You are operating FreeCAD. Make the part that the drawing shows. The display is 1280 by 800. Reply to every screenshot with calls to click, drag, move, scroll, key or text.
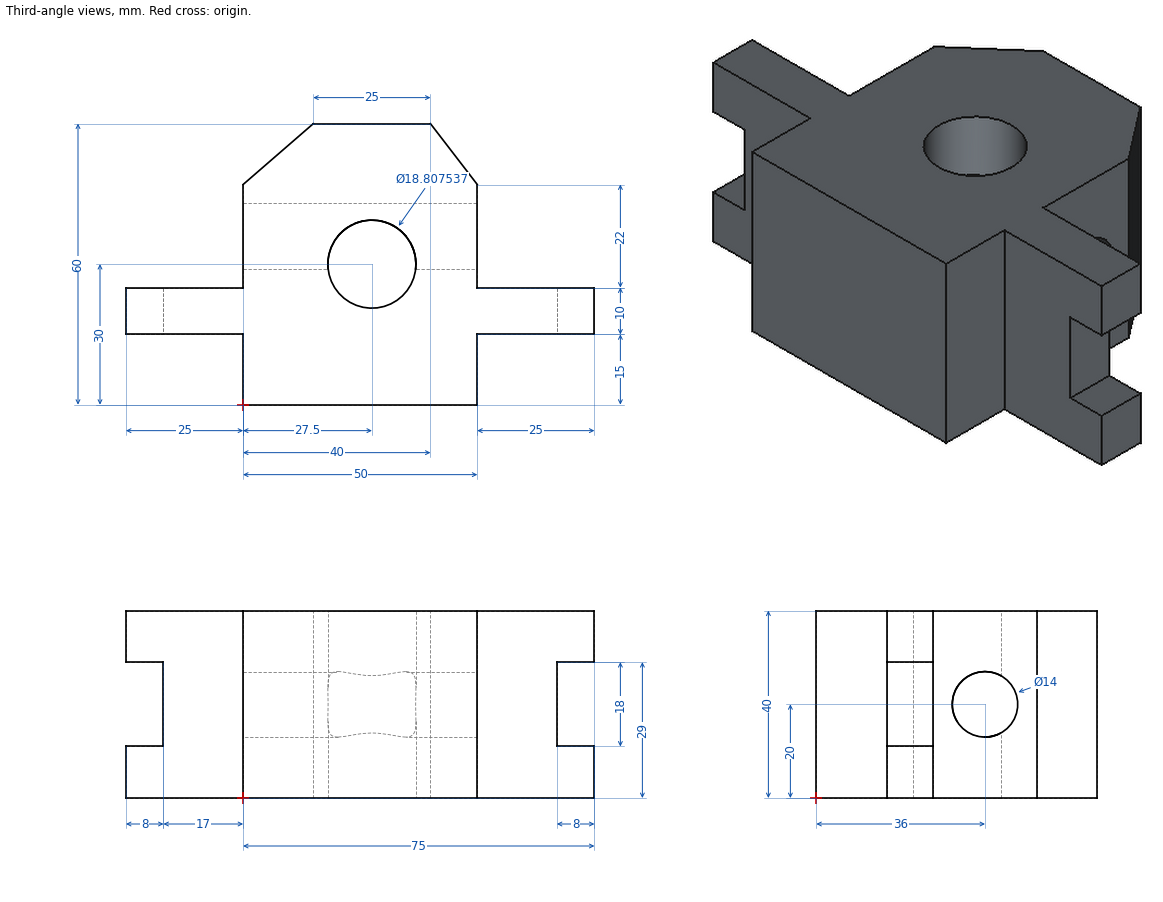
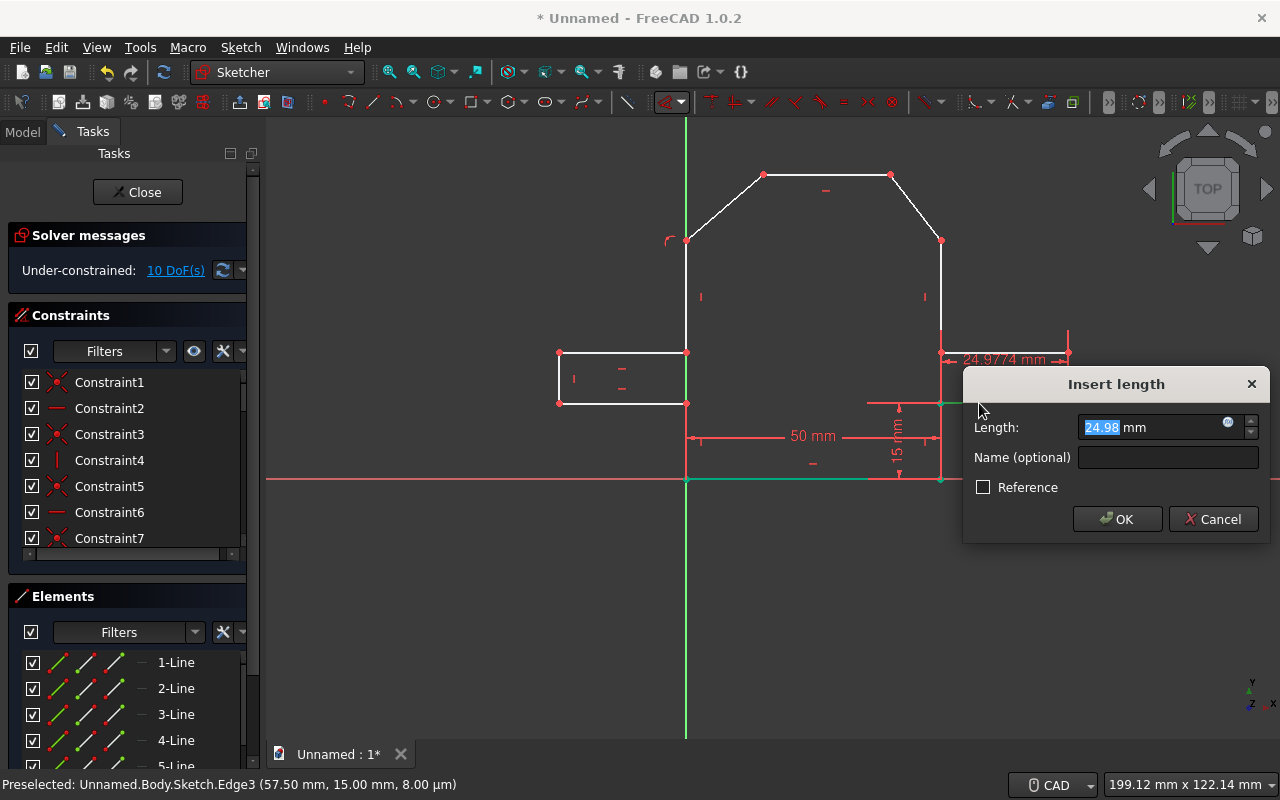
text(25)
key(Return)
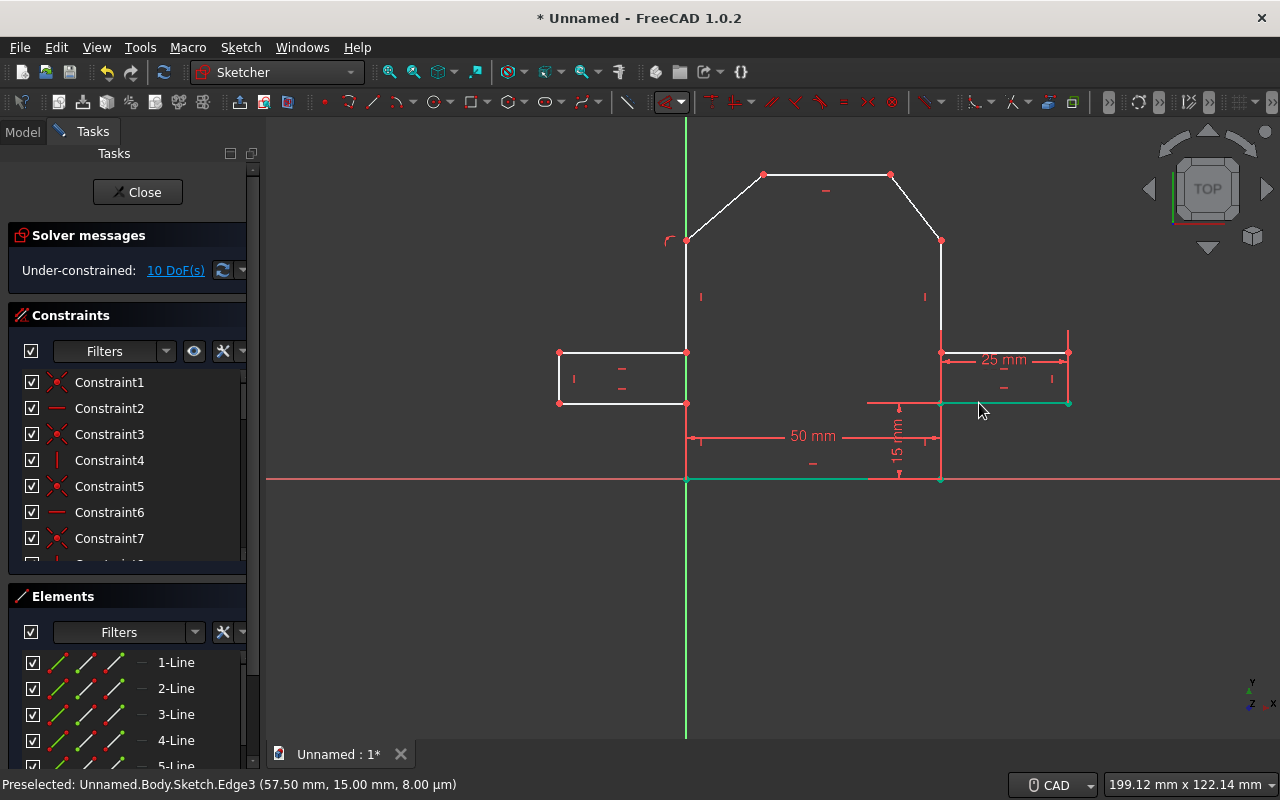
click(1068, 388)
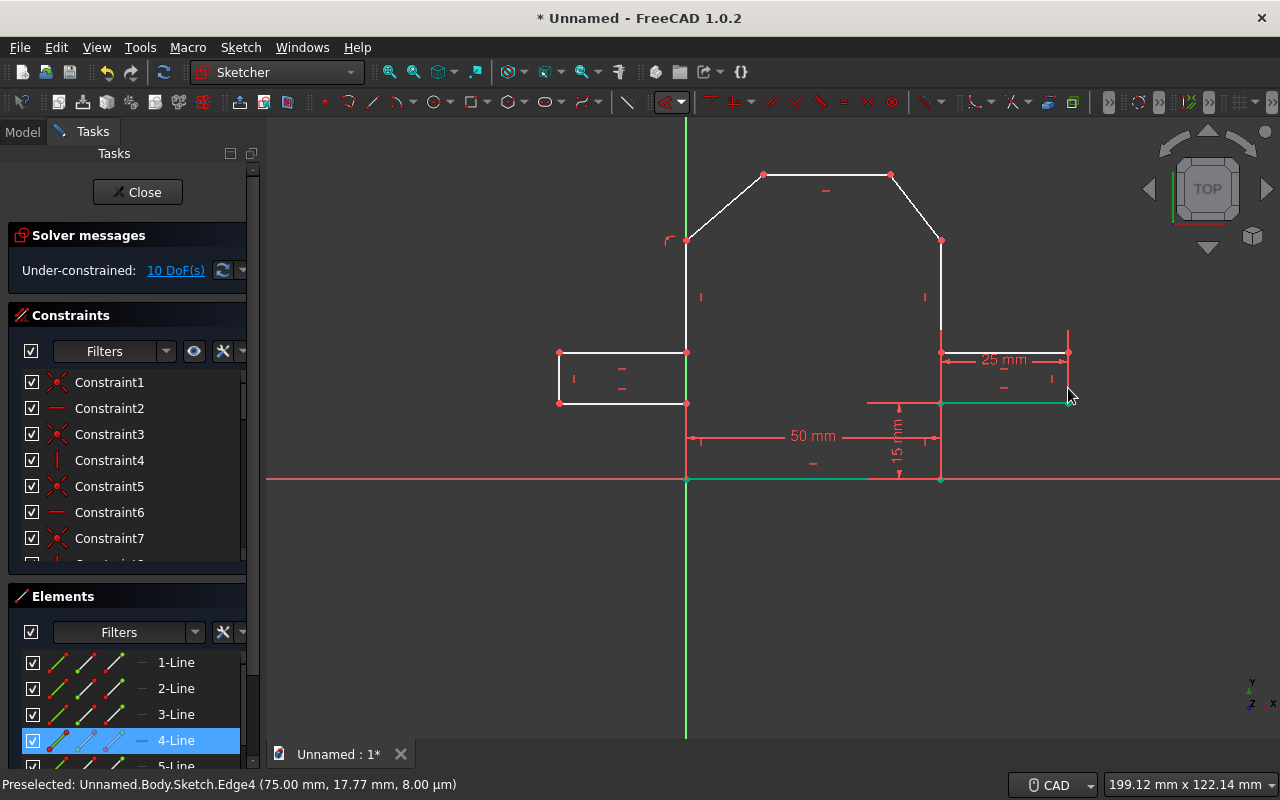
key(i)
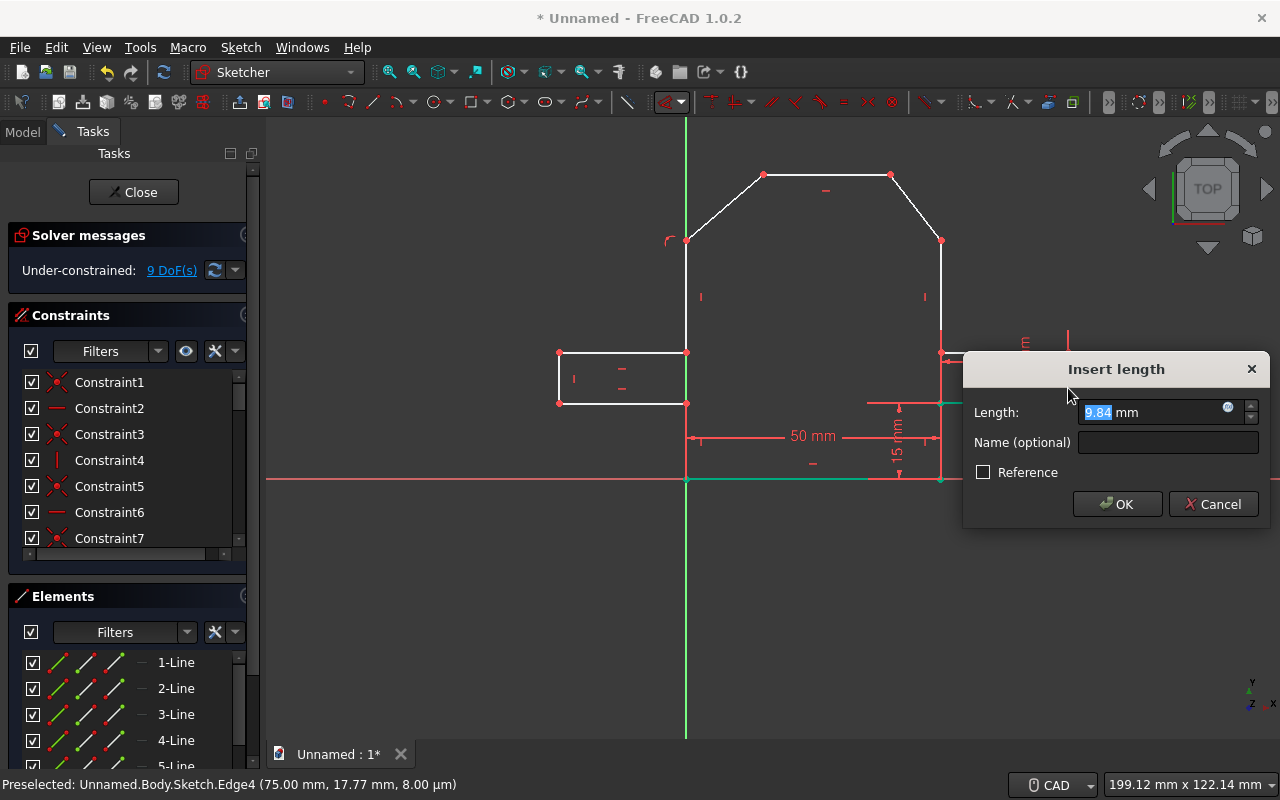
text(10)
key(Return)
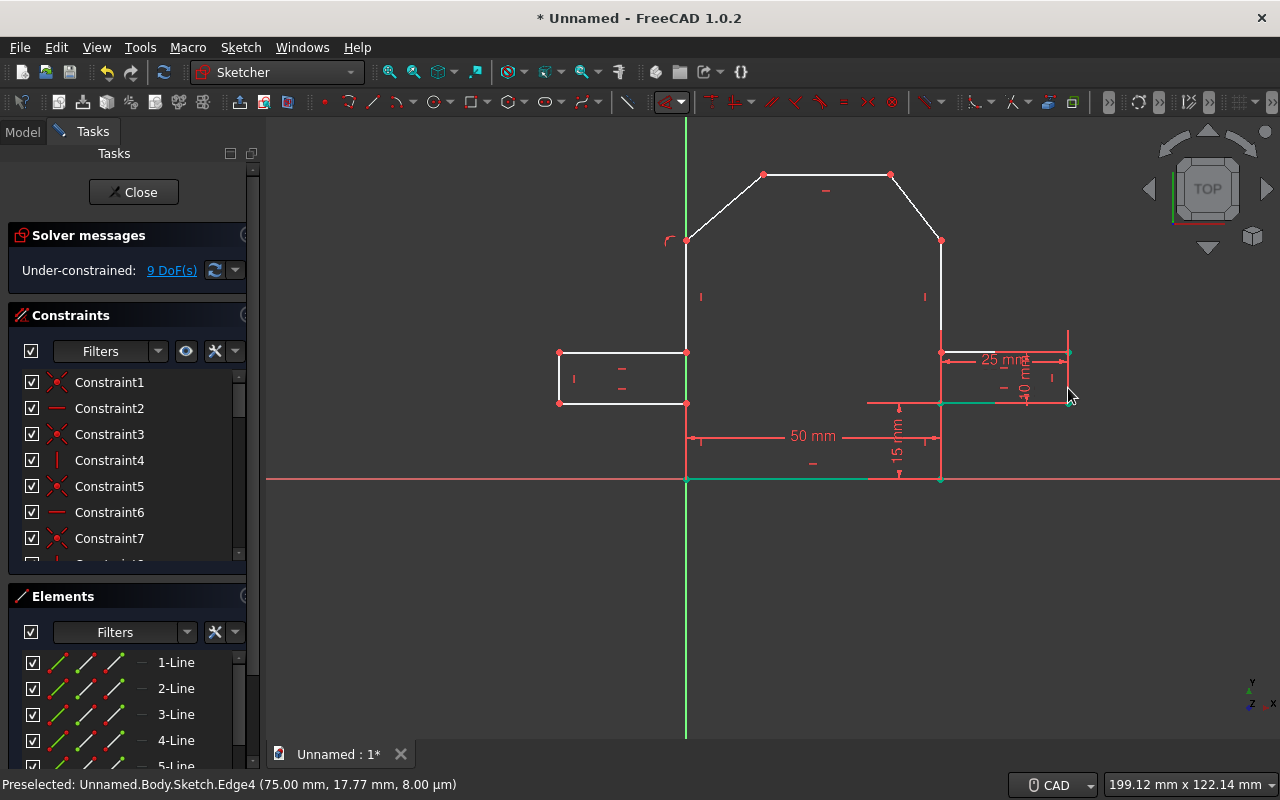
click(1030, 352)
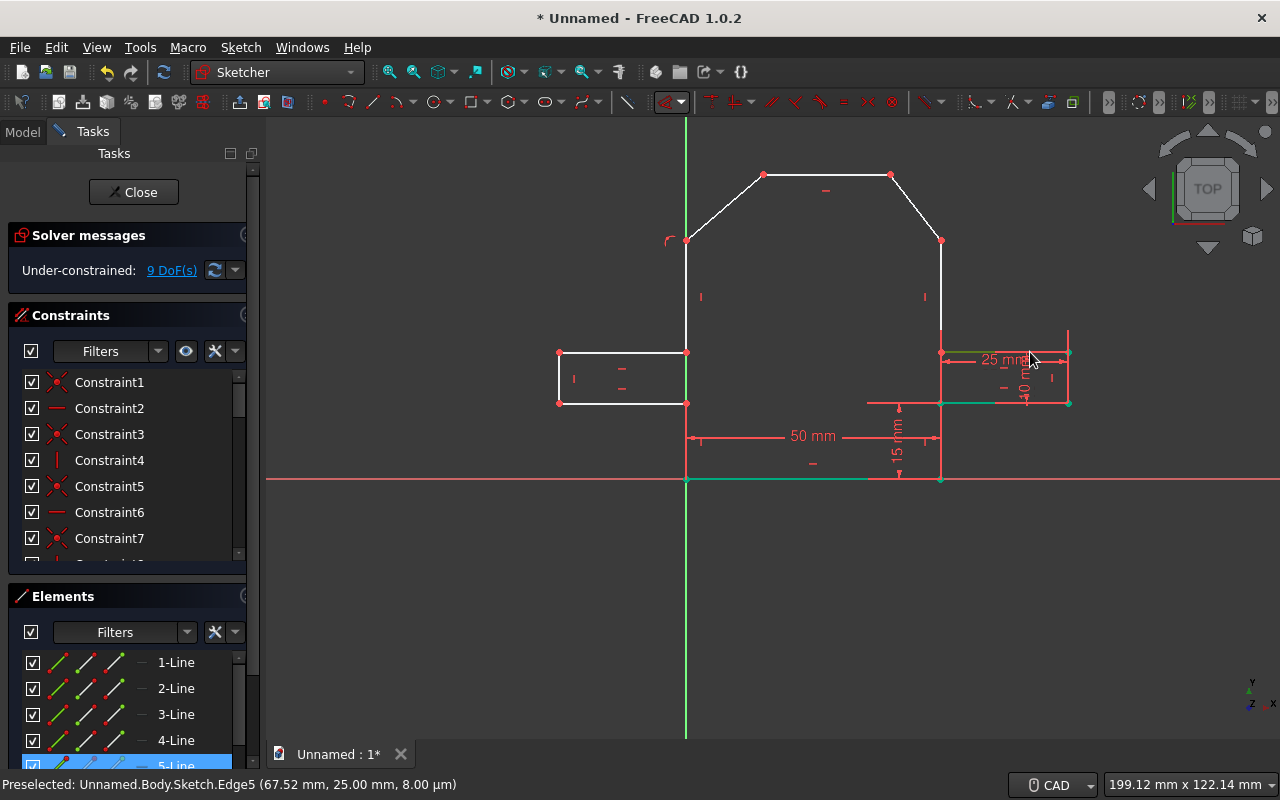
key(l)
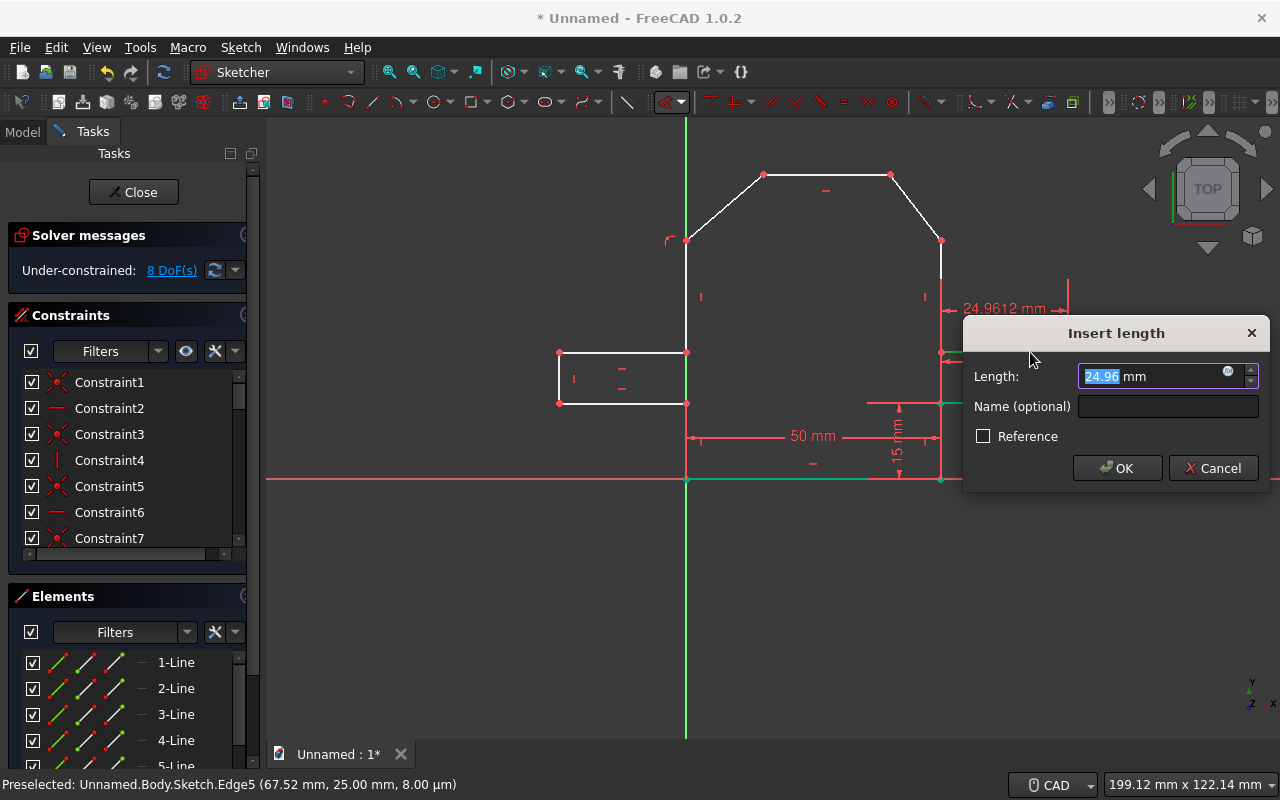
text(25)
key(Return)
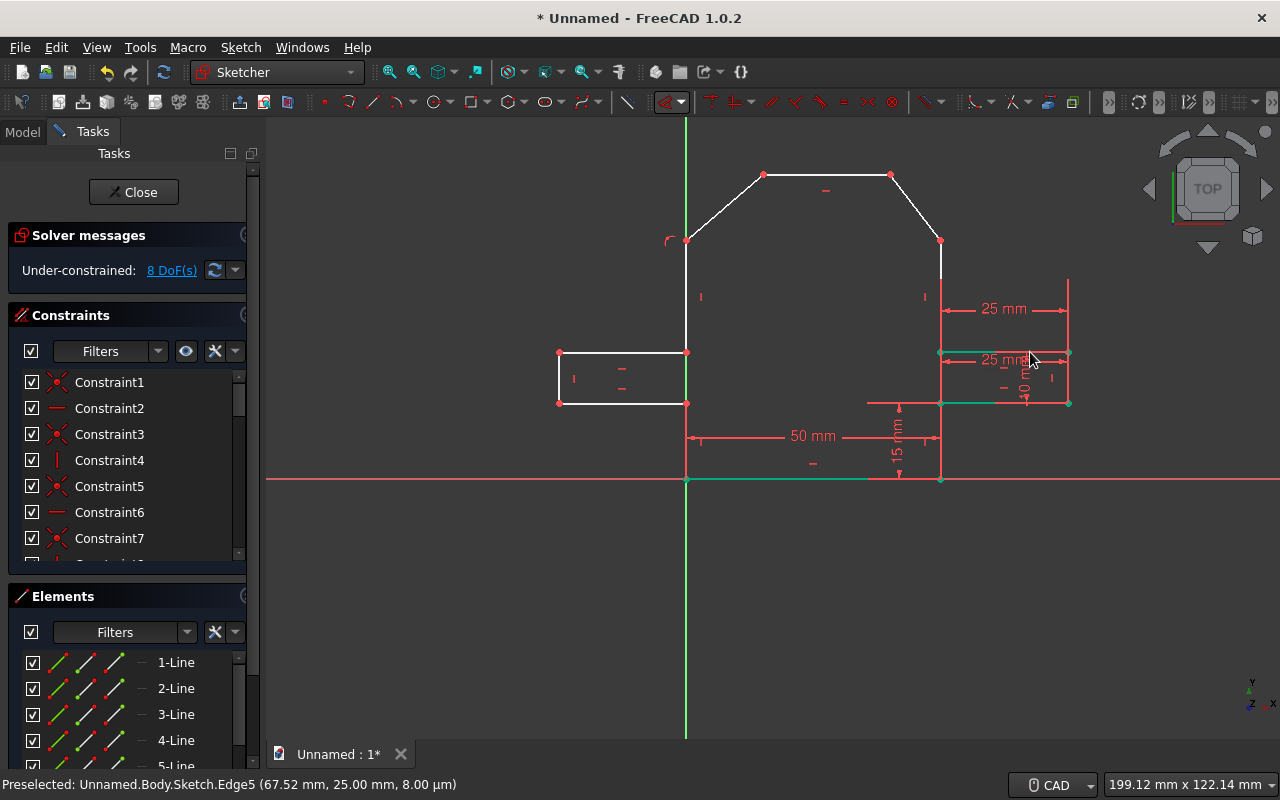
click(941, 319)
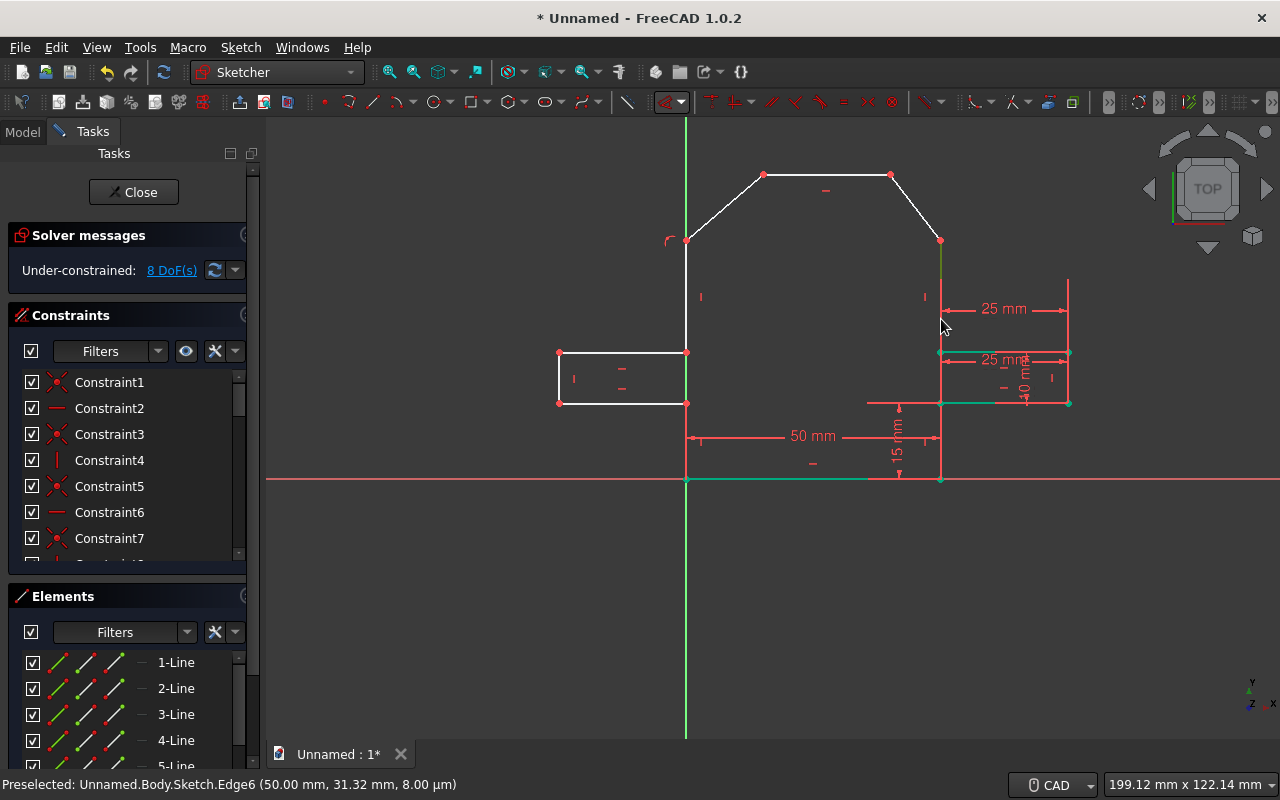
key(i)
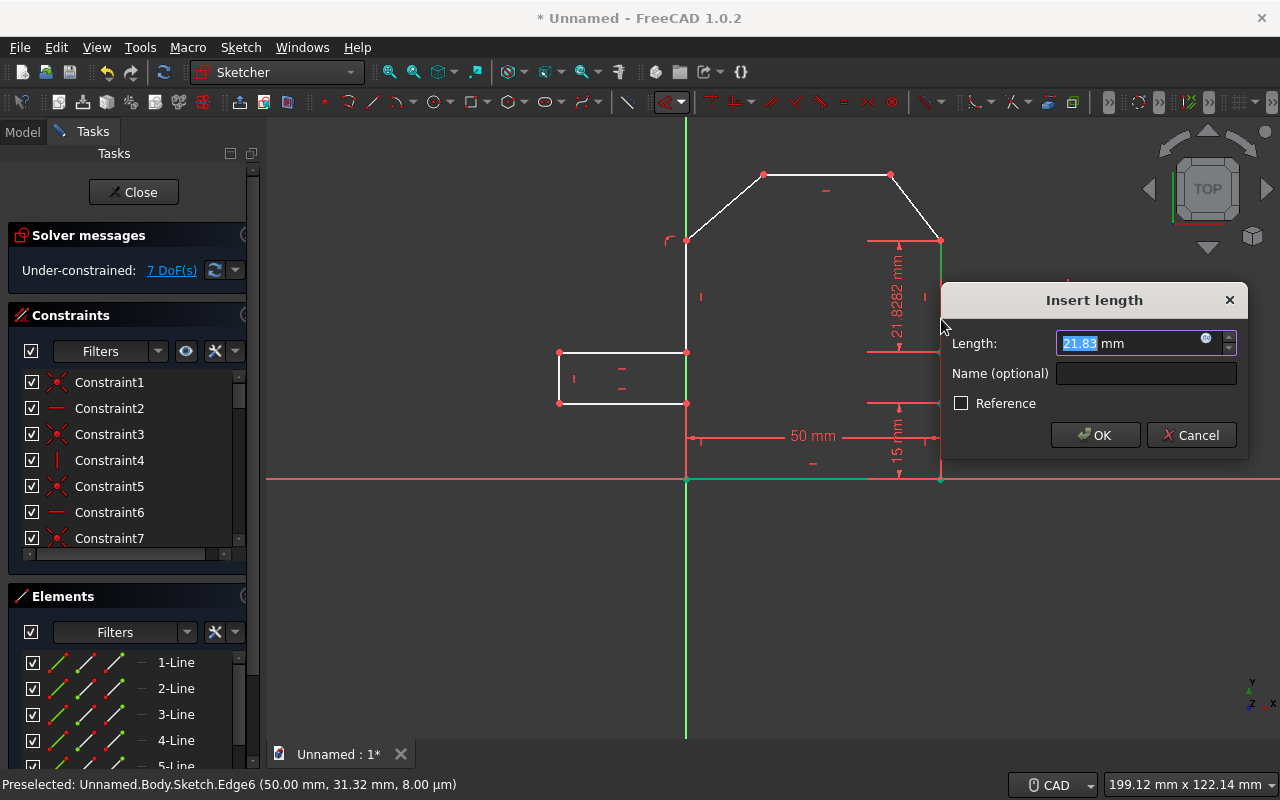
text(22)
key(Return)